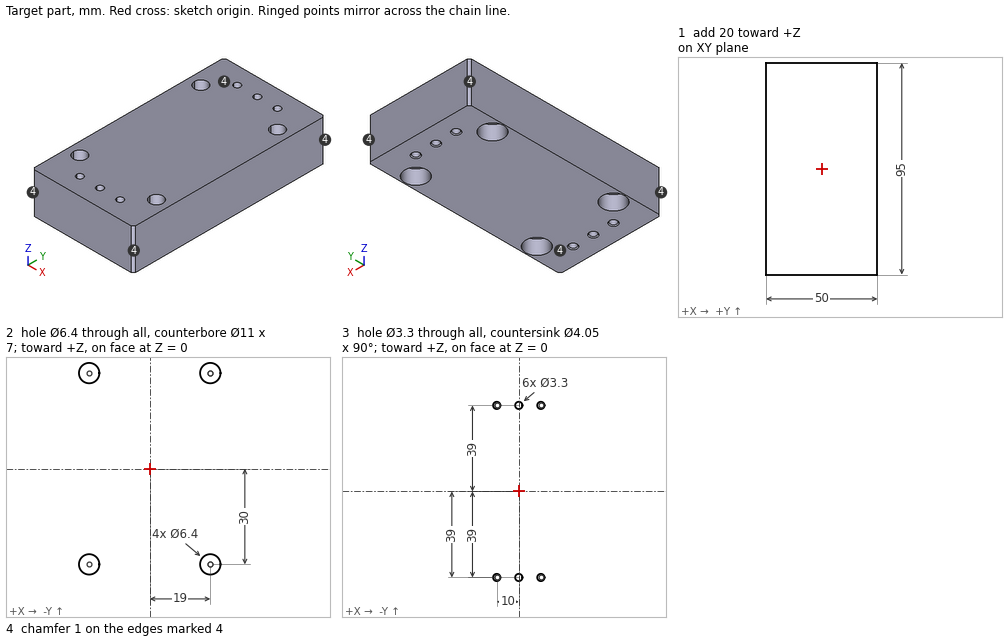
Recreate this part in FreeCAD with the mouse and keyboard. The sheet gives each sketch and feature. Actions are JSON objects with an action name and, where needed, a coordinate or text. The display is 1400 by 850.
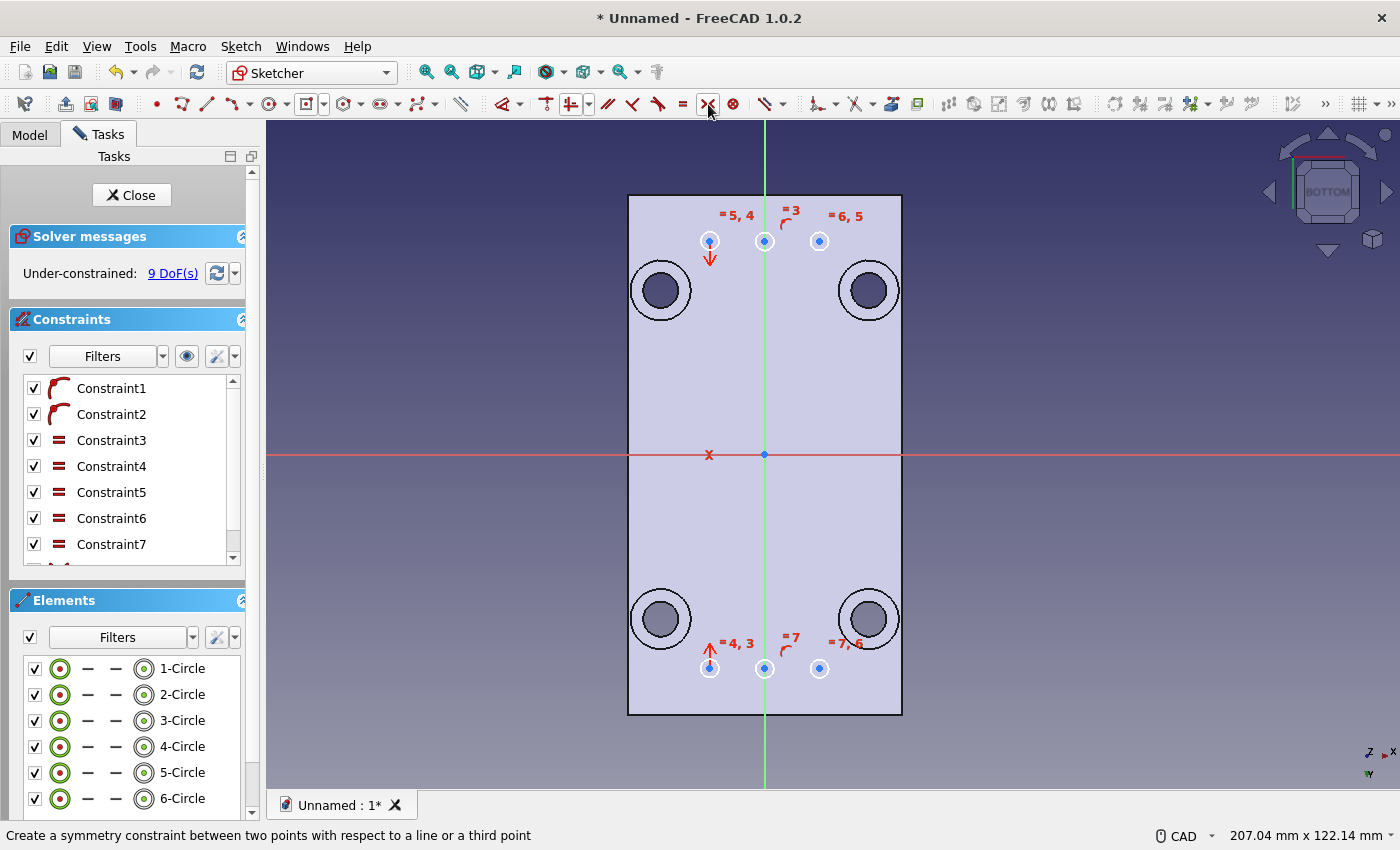
{"action": "left_click", "coordinate": [710, 241]}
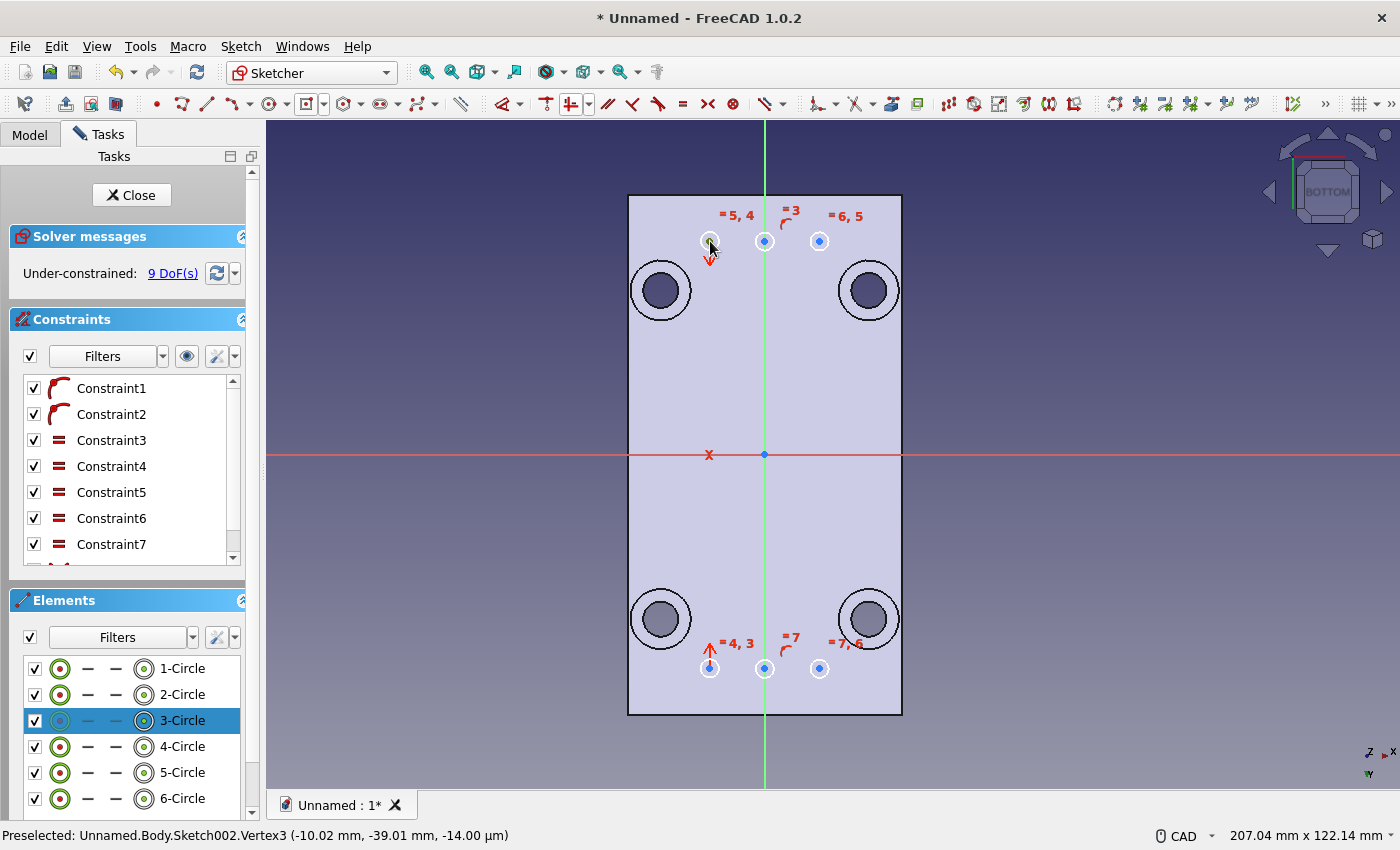
{"action": "left_click", "coordinate": [820, 241]}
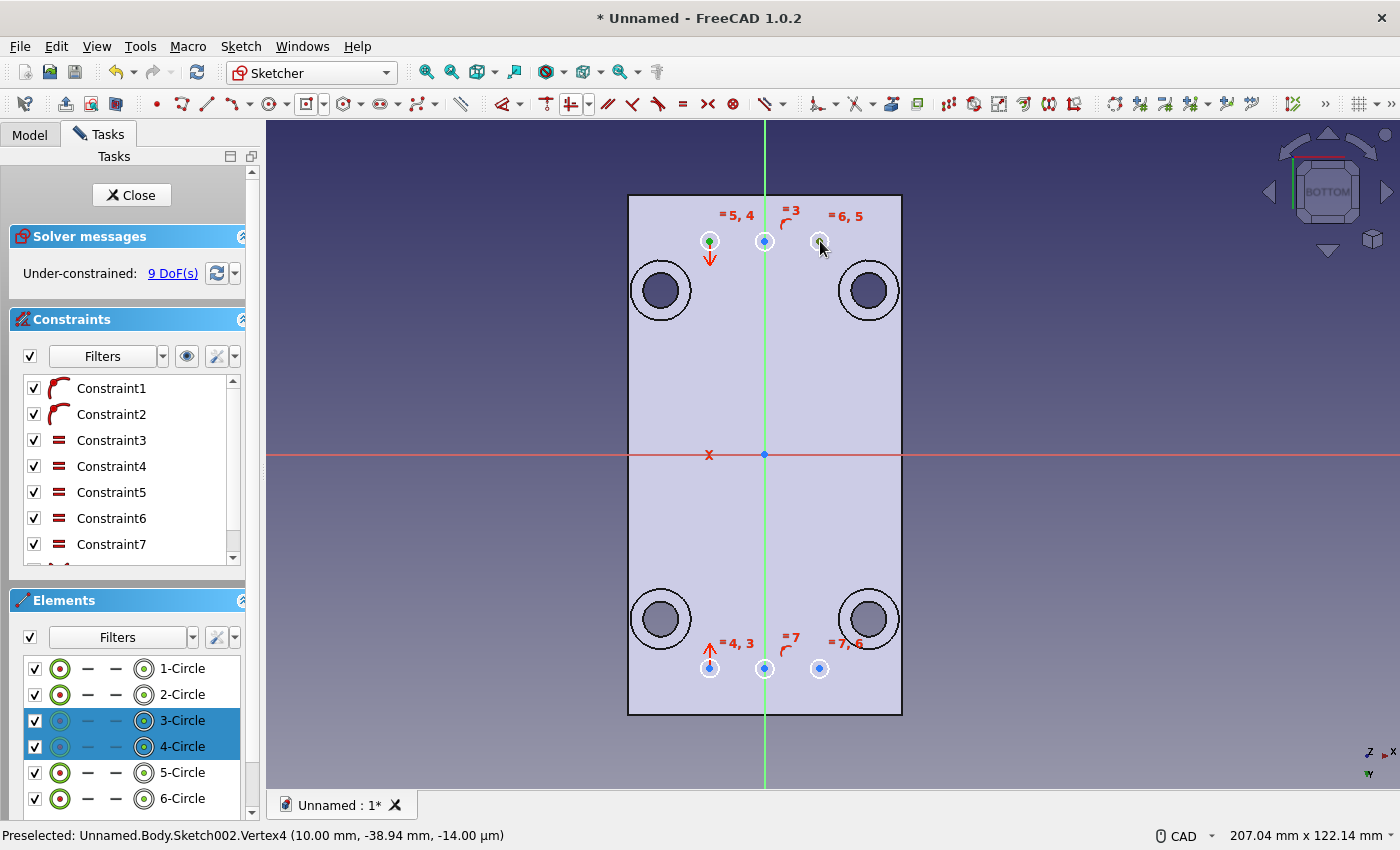
{"action": "left_click", "coordinate": [765, 717]}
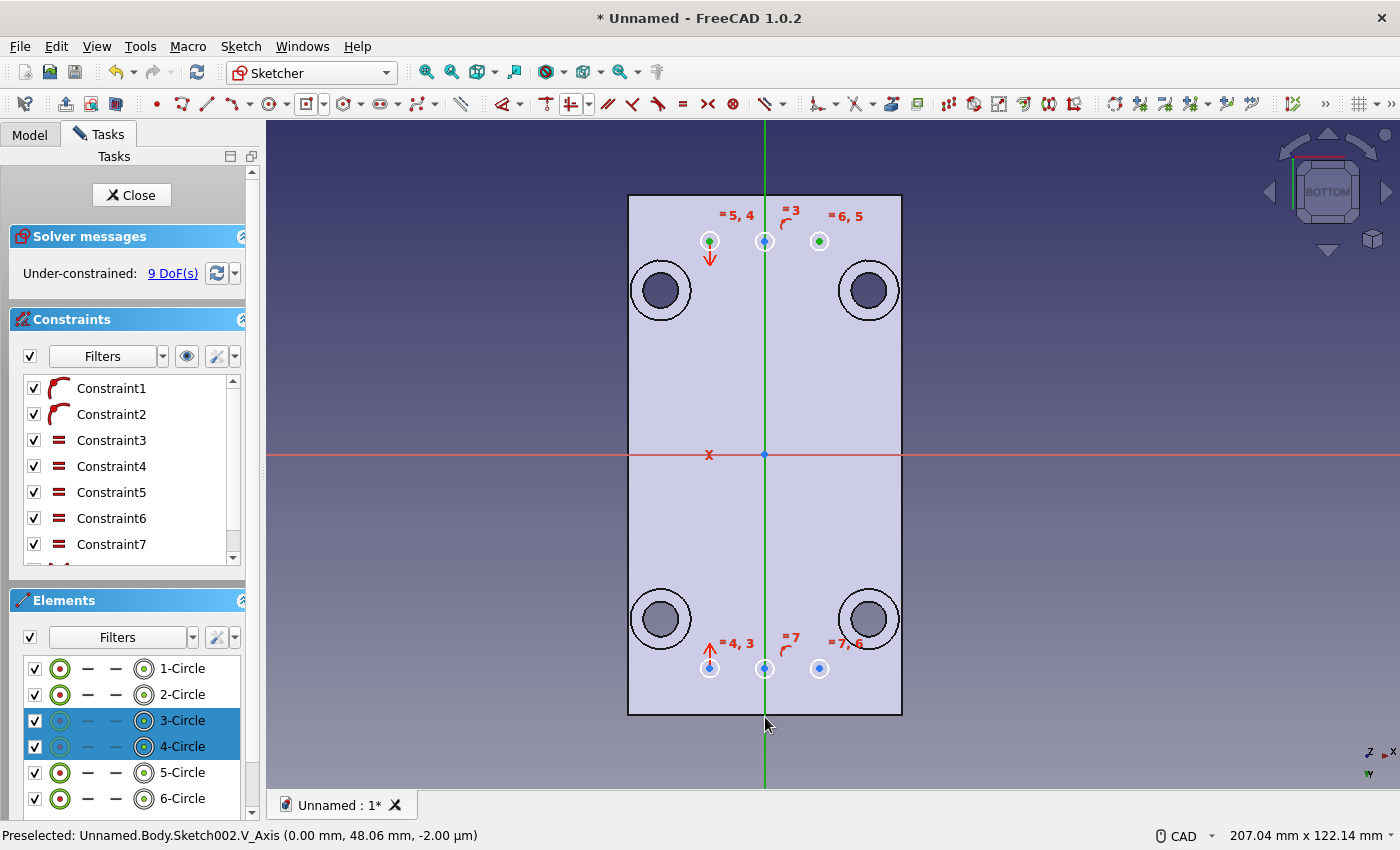
{"action": "left_click", "coordinate": [708, 104]}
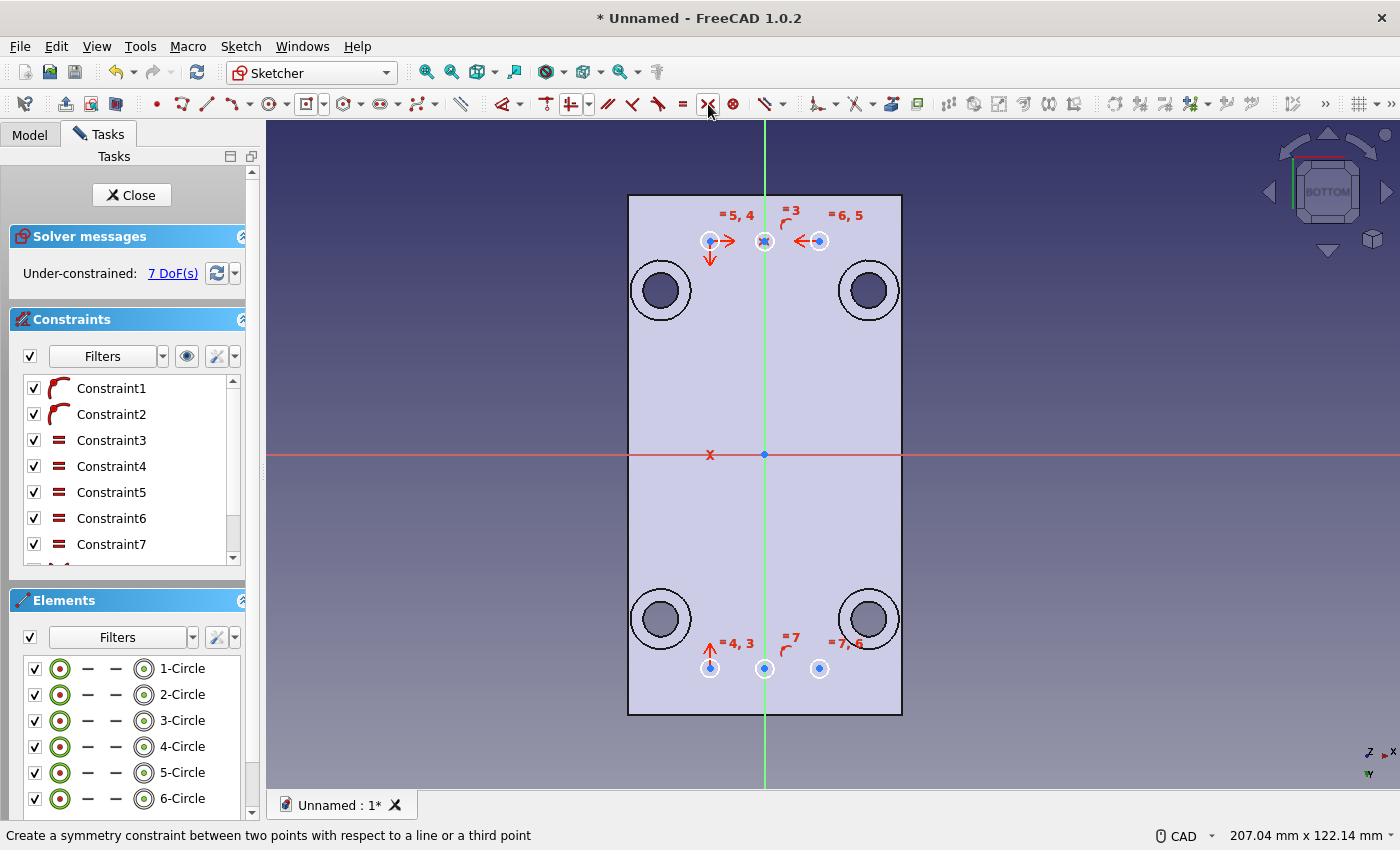
{"action": "left_click", "coordinate": [710, 668]}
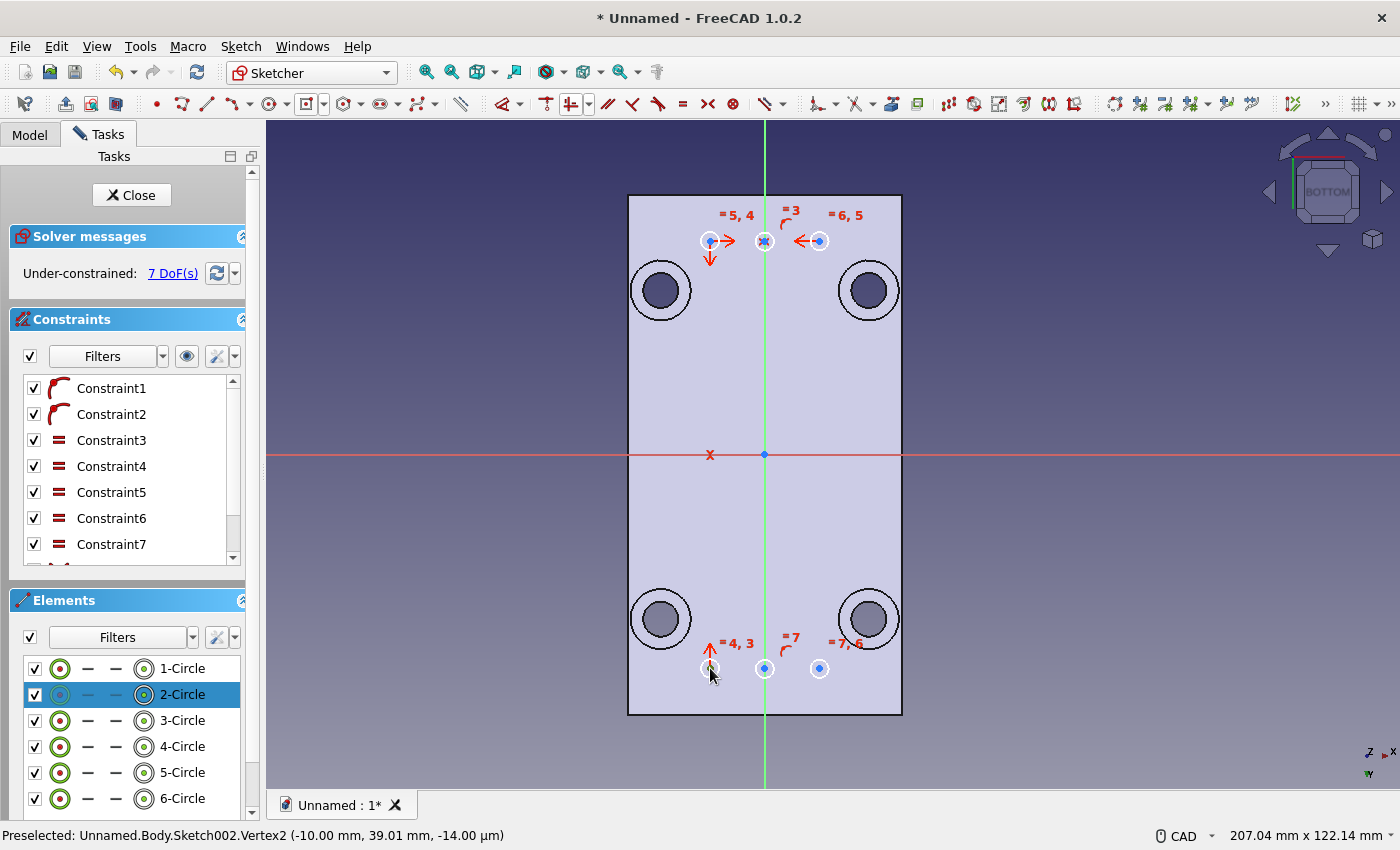
{"action": "left_click", "coordinate": [820, 669]}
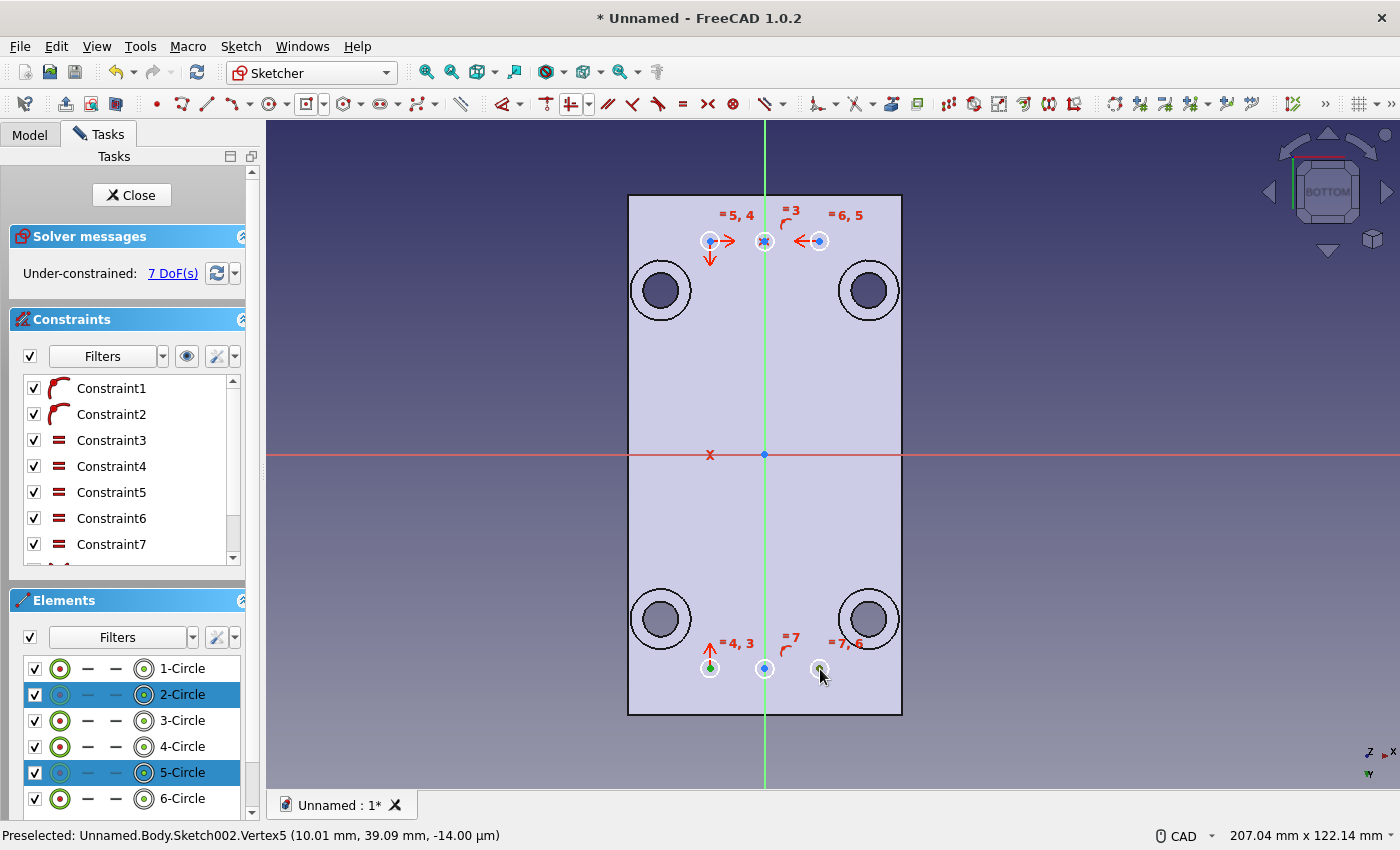
{"action": "left_click", "coordinate": [765, 717]}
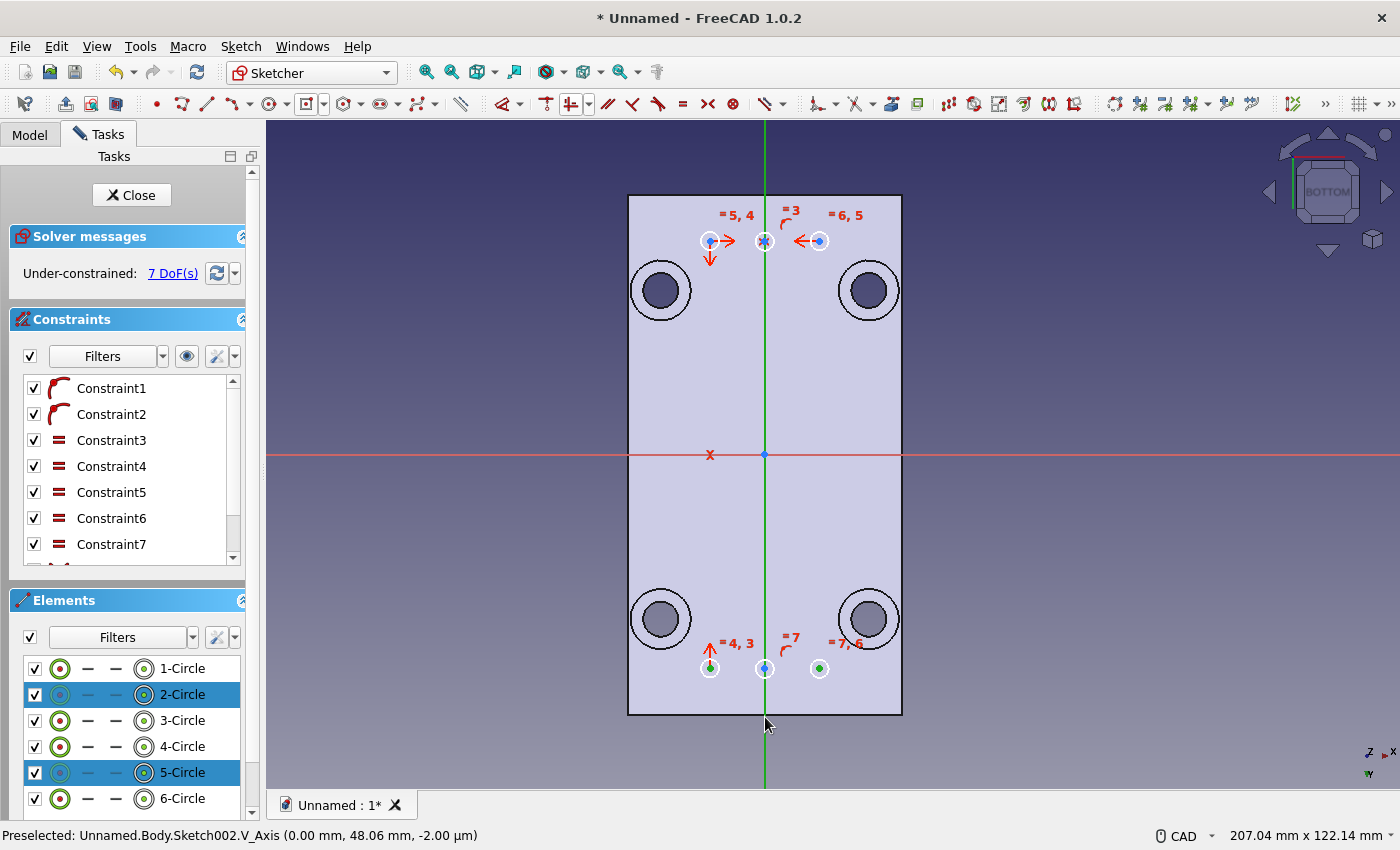
{"action": "left_click", "coordinate": [708, 104]}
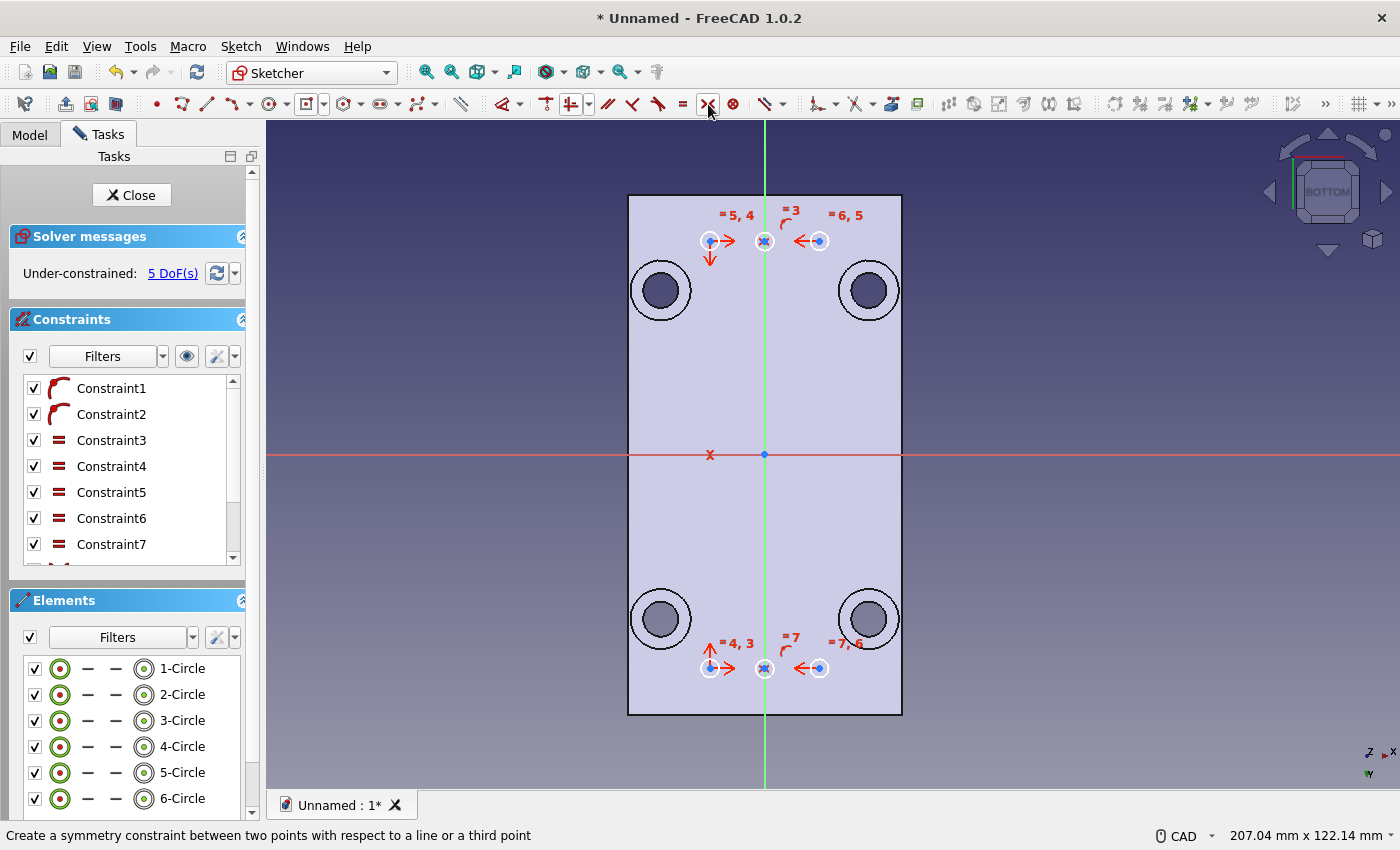
{"action": "left_click", "coordinate": [502, 104]}